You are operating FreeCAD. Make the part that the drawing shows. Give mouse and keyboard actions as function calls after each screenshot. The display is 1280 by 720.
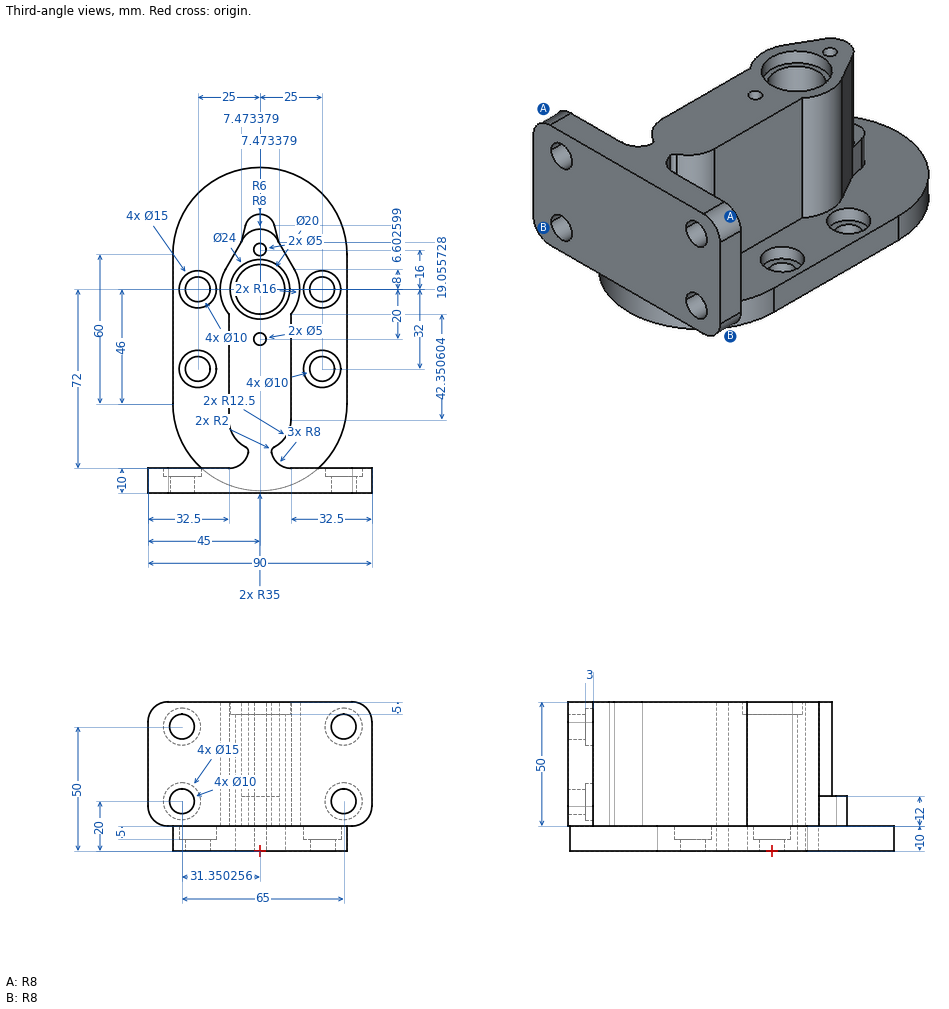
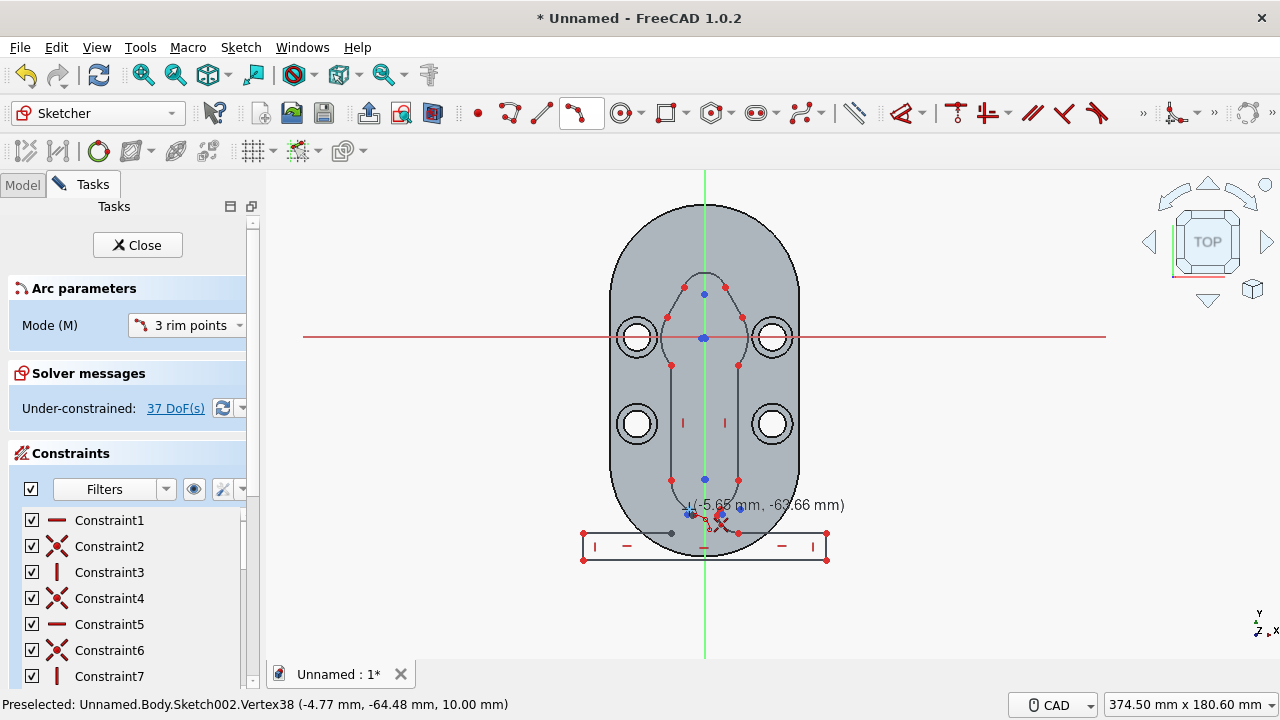
scroll(692, 515, up, 6)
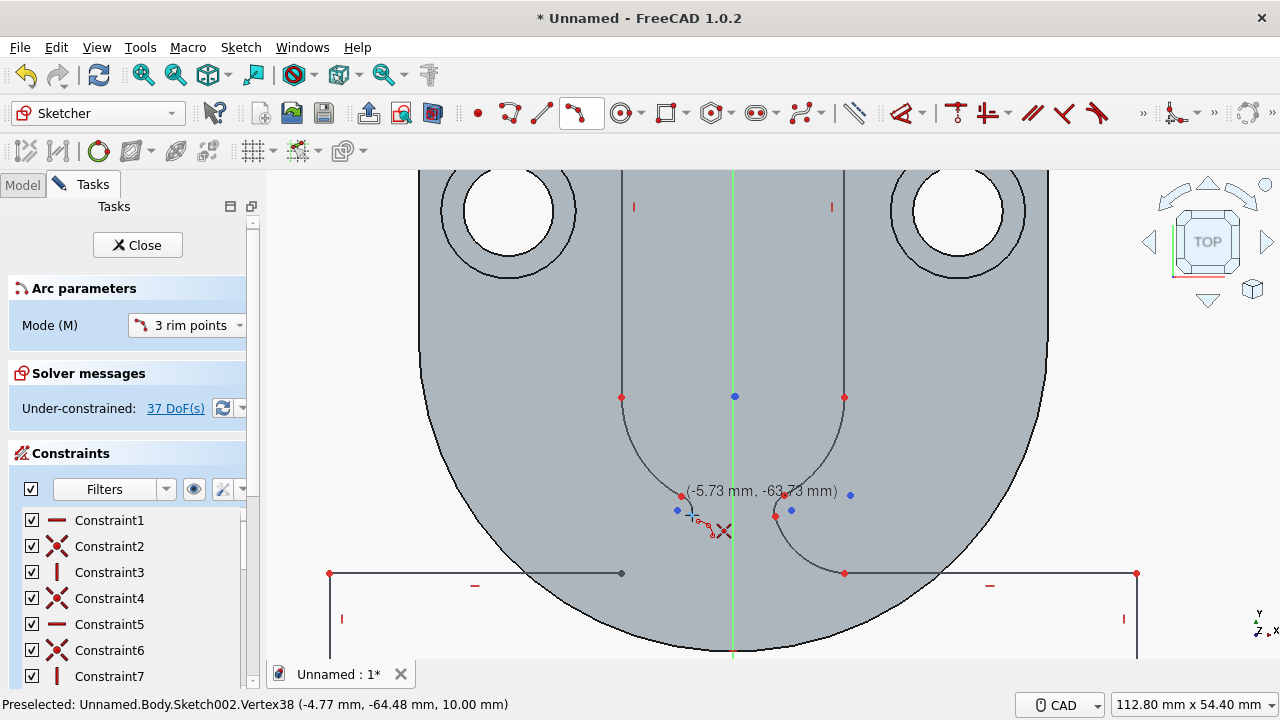
click(691, 515)
click(622, 573)
click(666, 555)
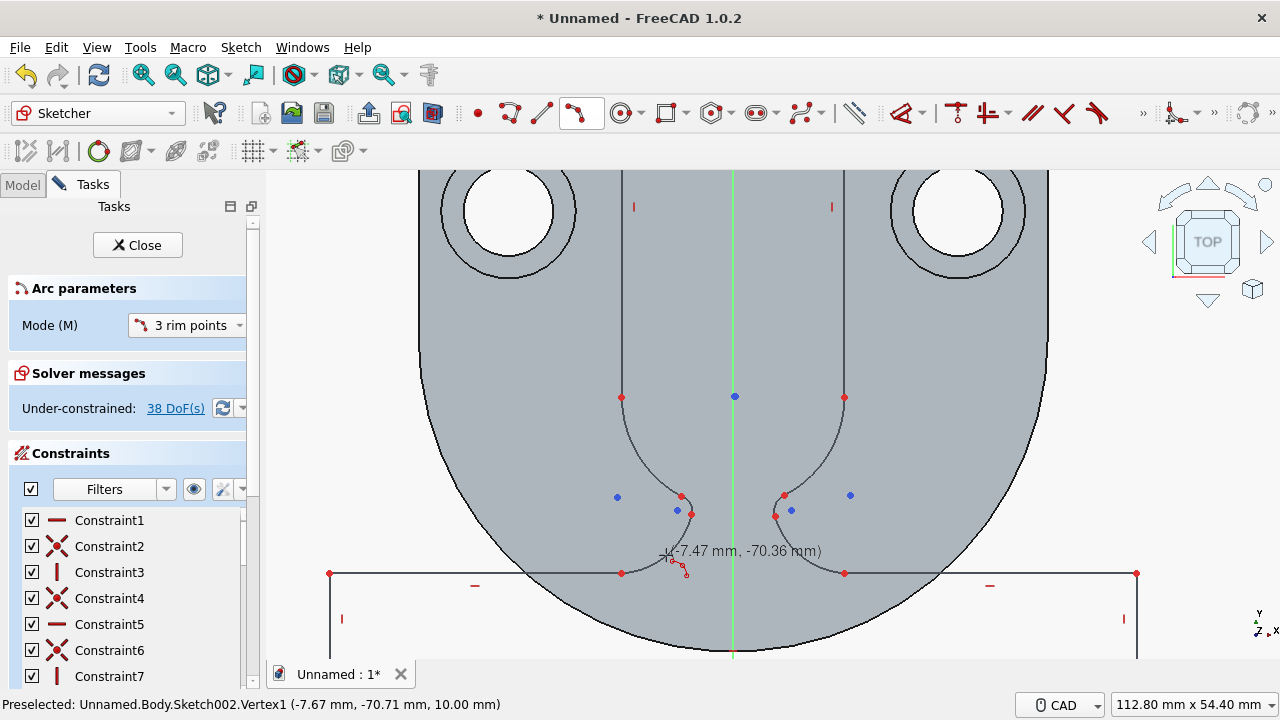
click(622, 114)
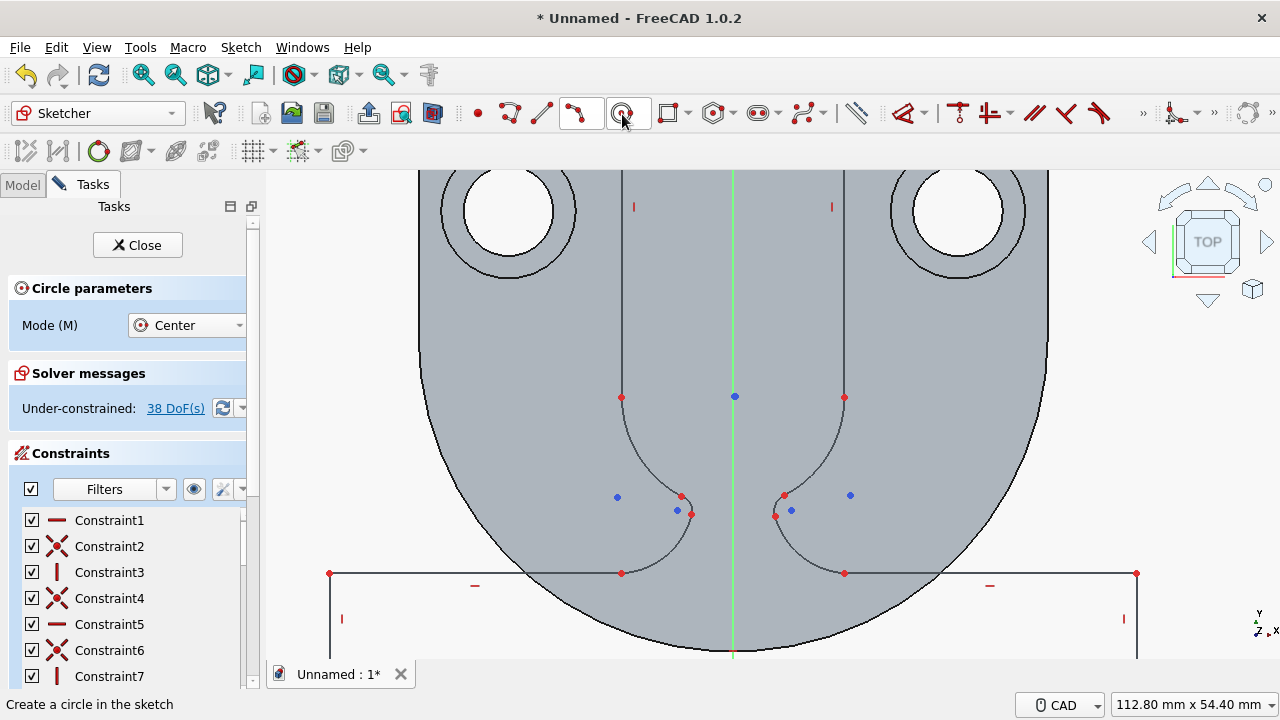
scroll(692, 514, down, 6)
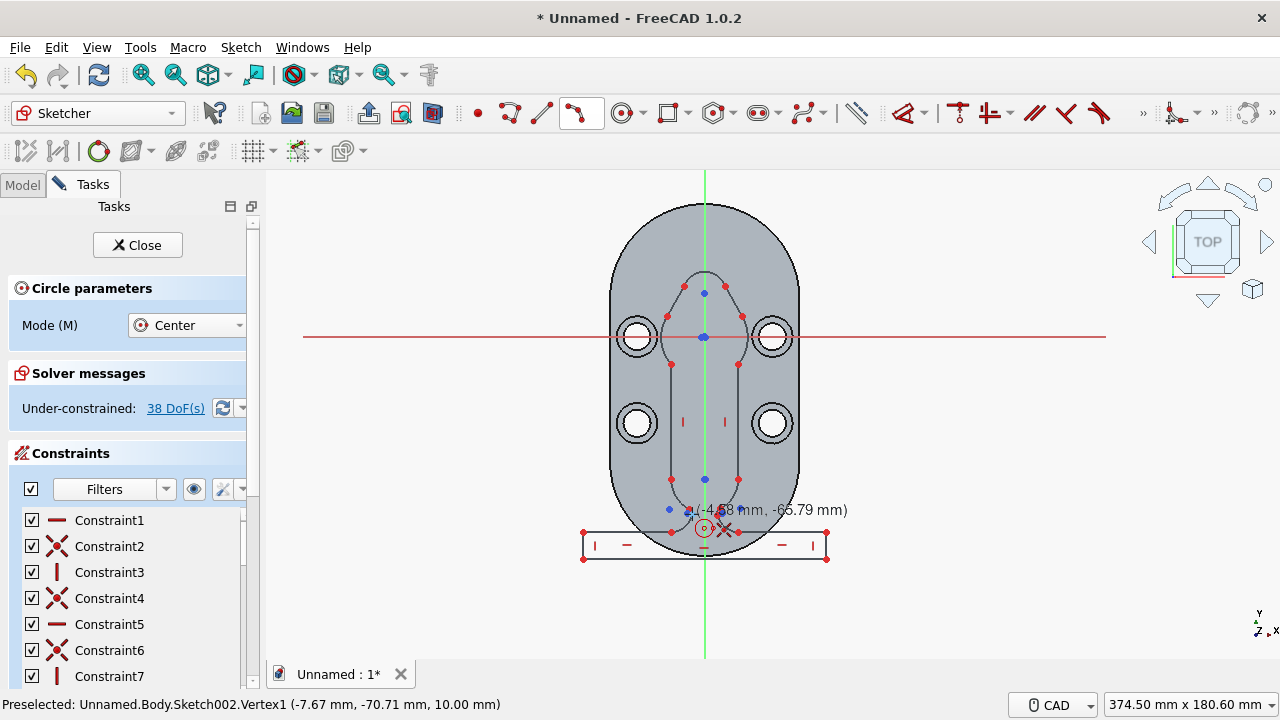
scroll(705, 391, up, 7)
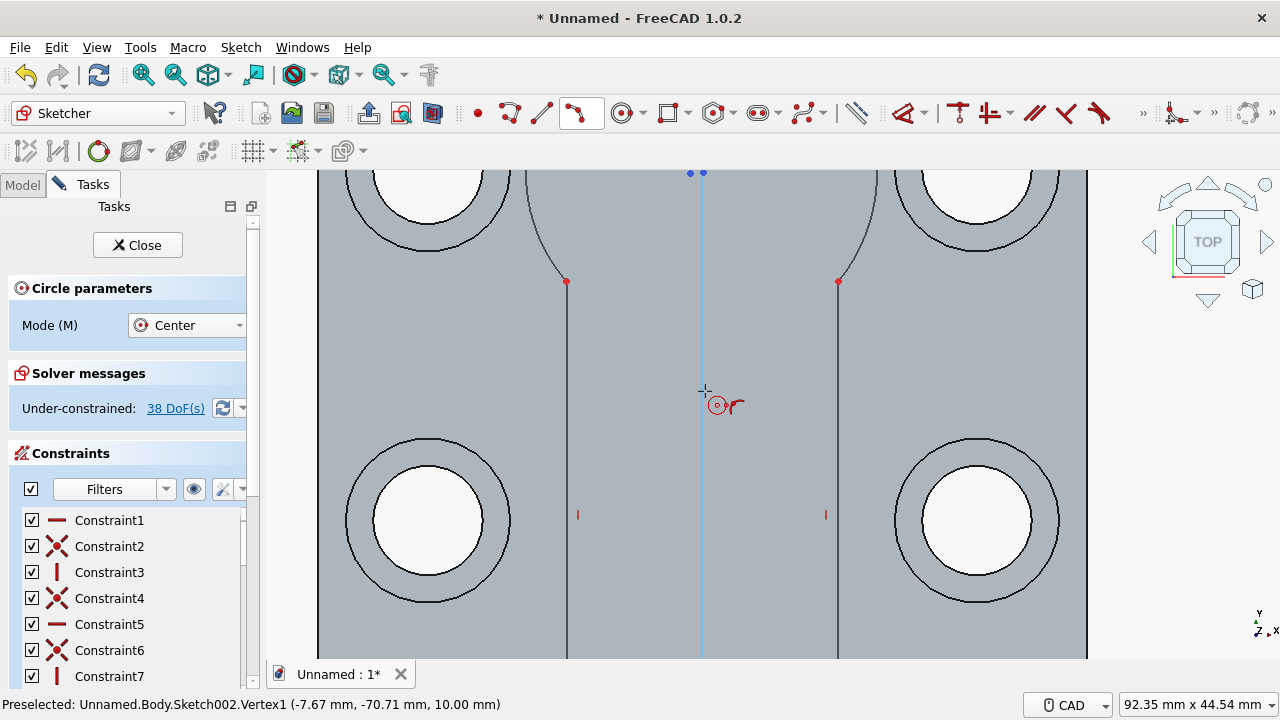
scroll(705, 391, down, 7)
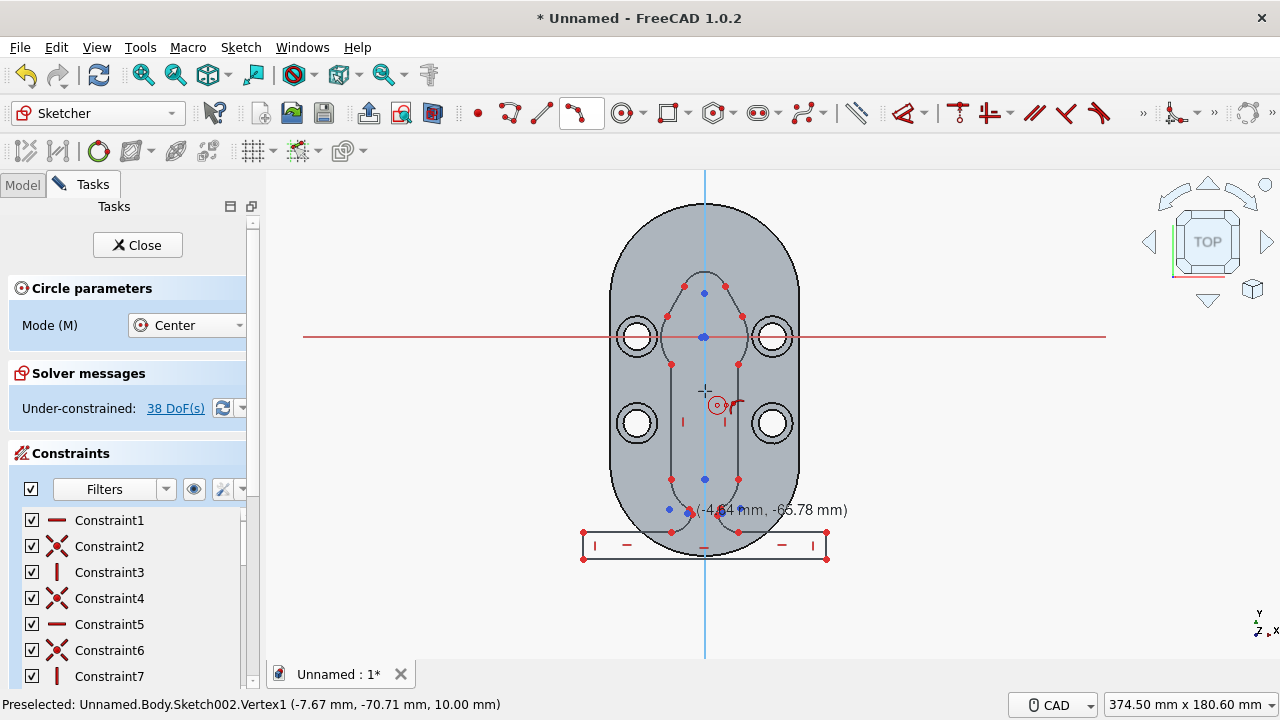
click(705, 391)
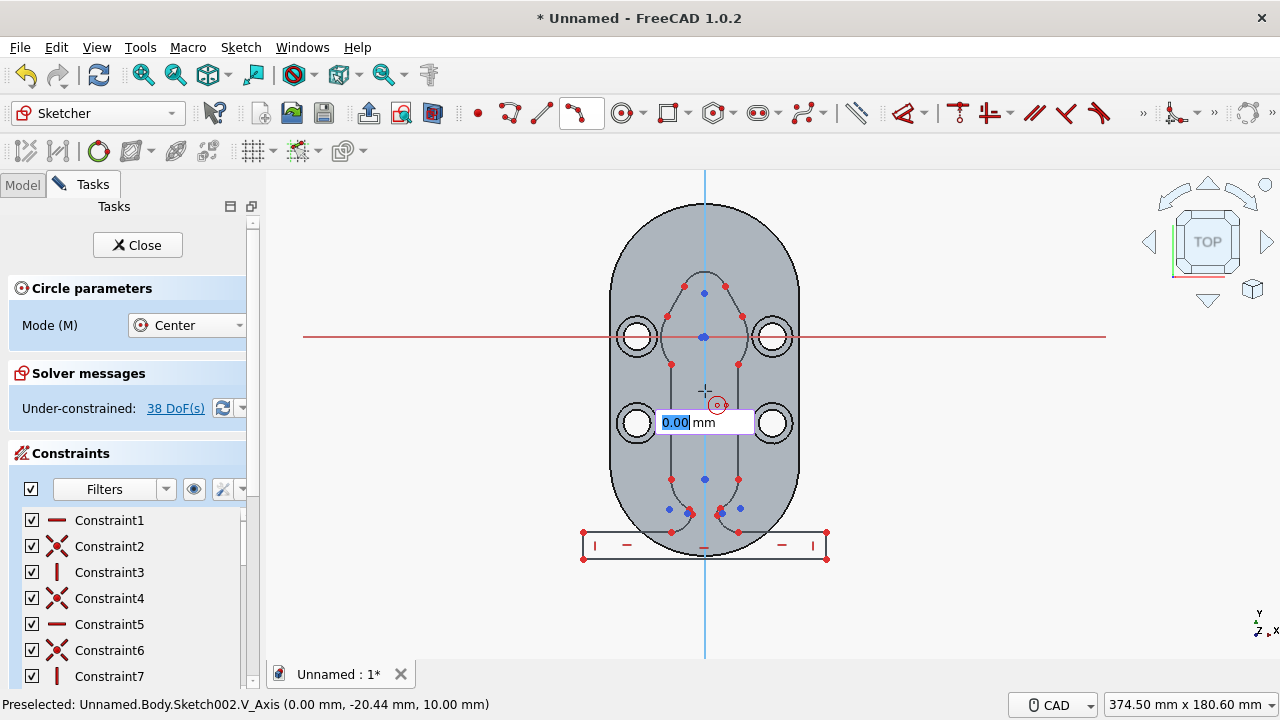
scroll(711, 388, up, 5)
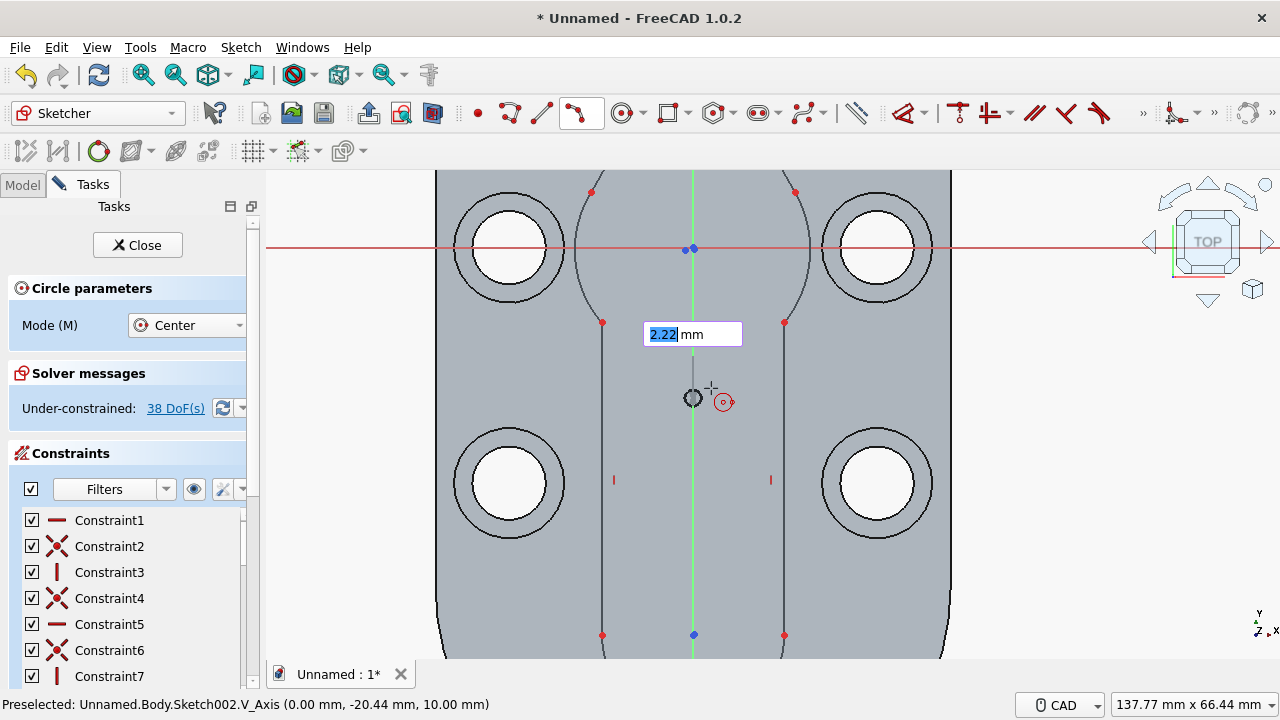
click(710, 389)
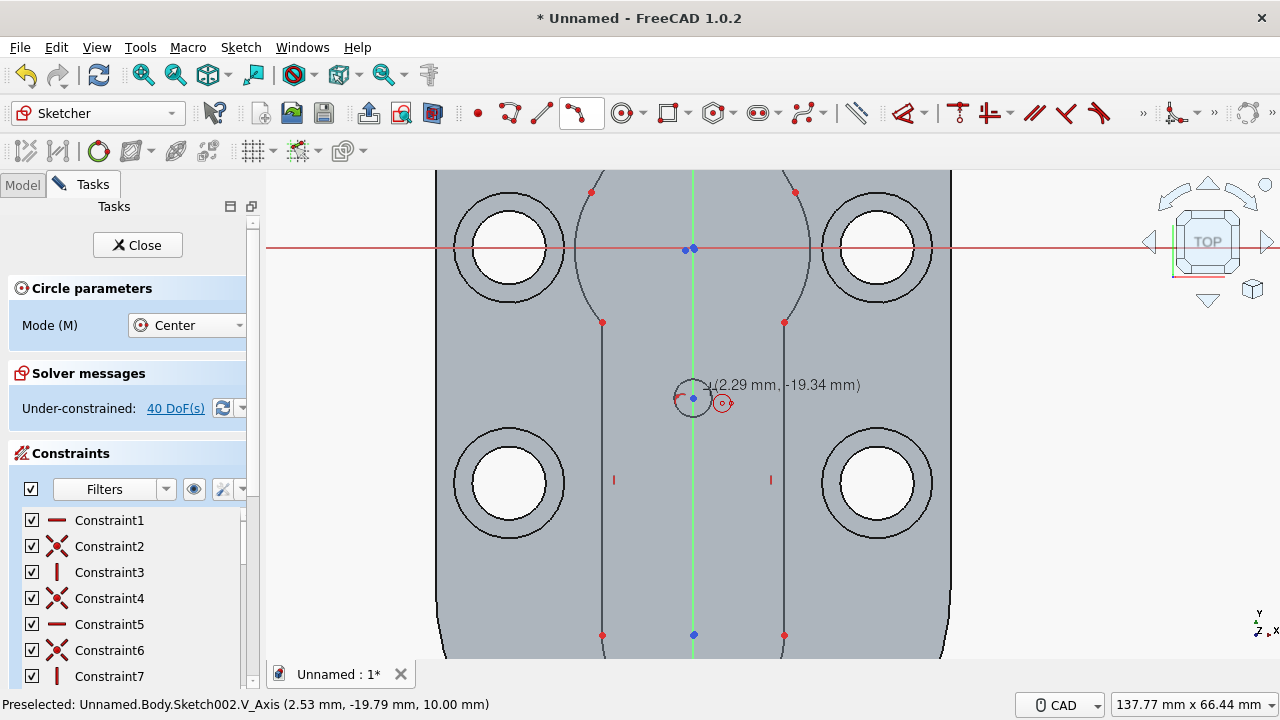
click(693, 248)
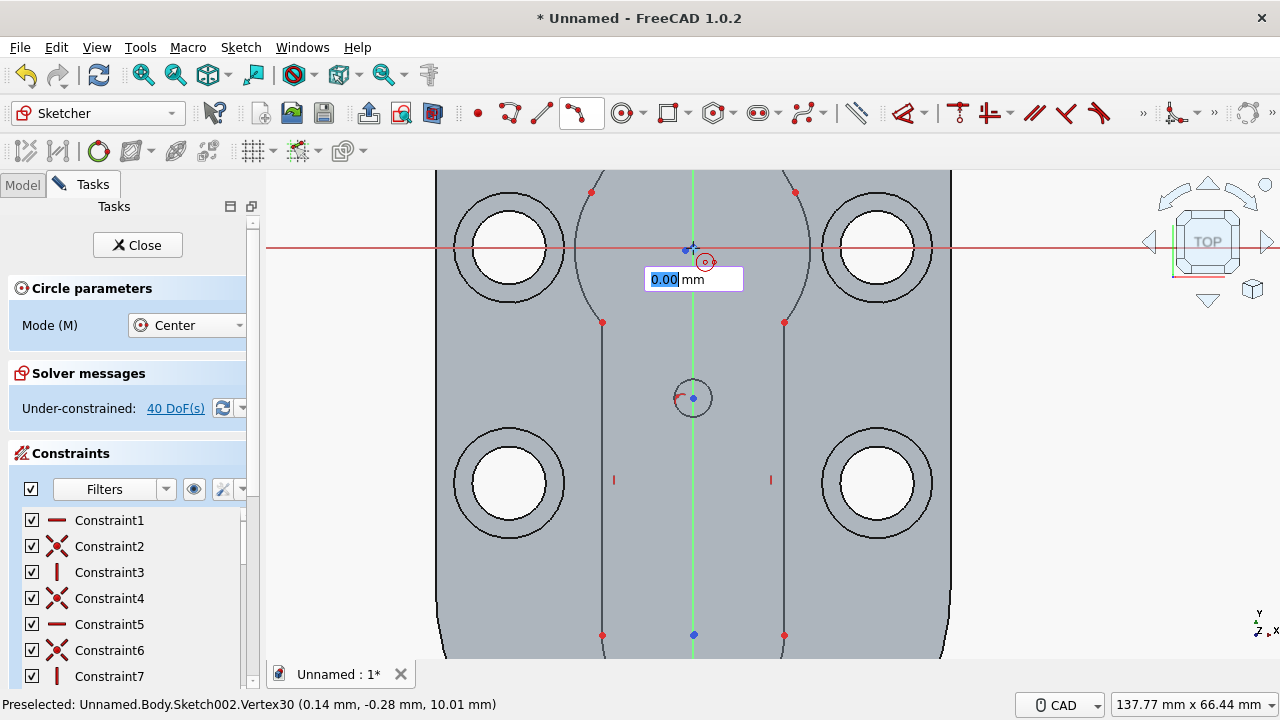
scroll(711, 388, down, 5)